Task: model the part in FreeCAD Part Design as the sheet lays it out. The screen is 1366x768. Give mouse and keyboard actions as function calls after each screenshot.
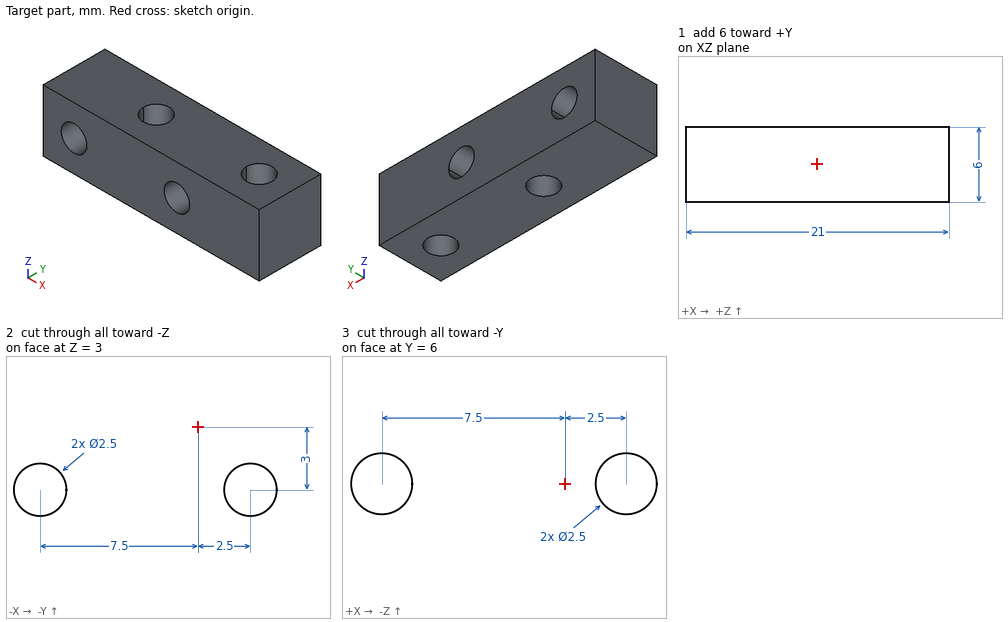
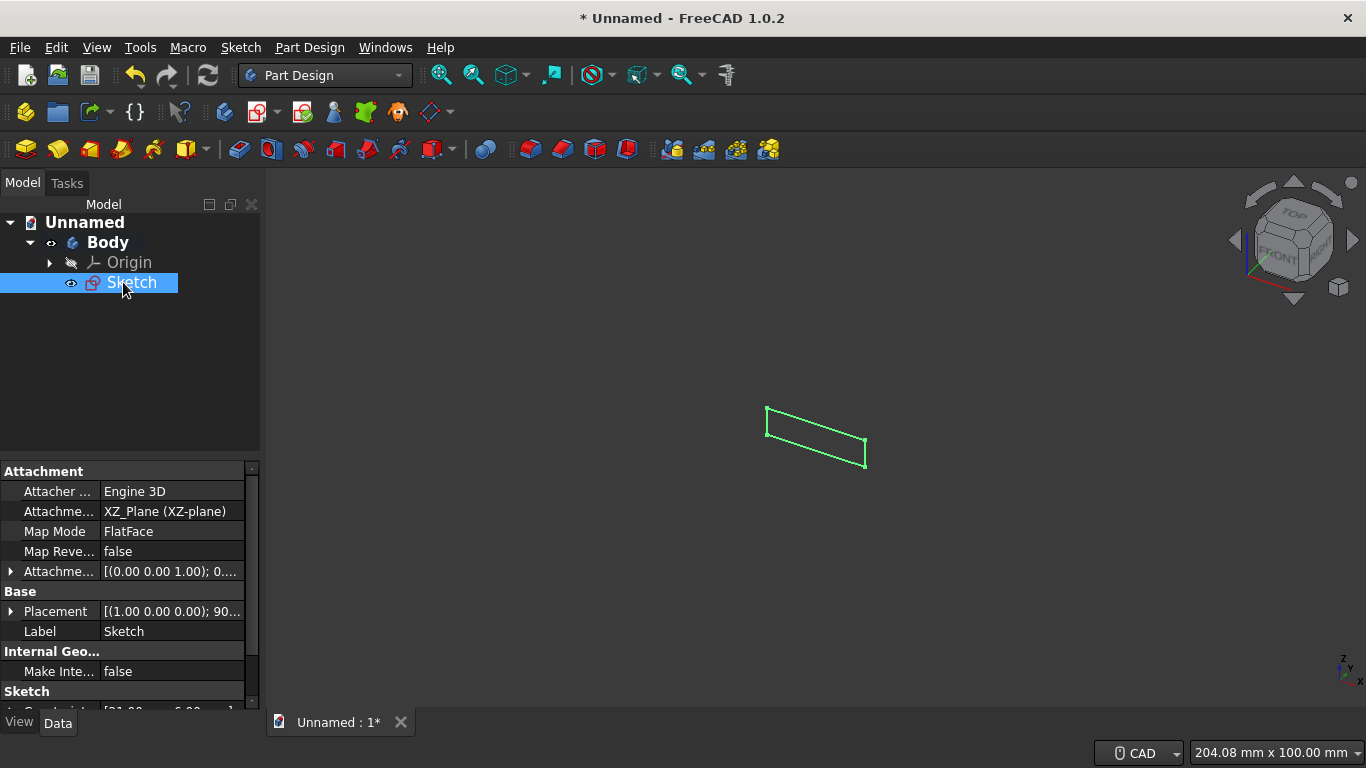
click(26, 150)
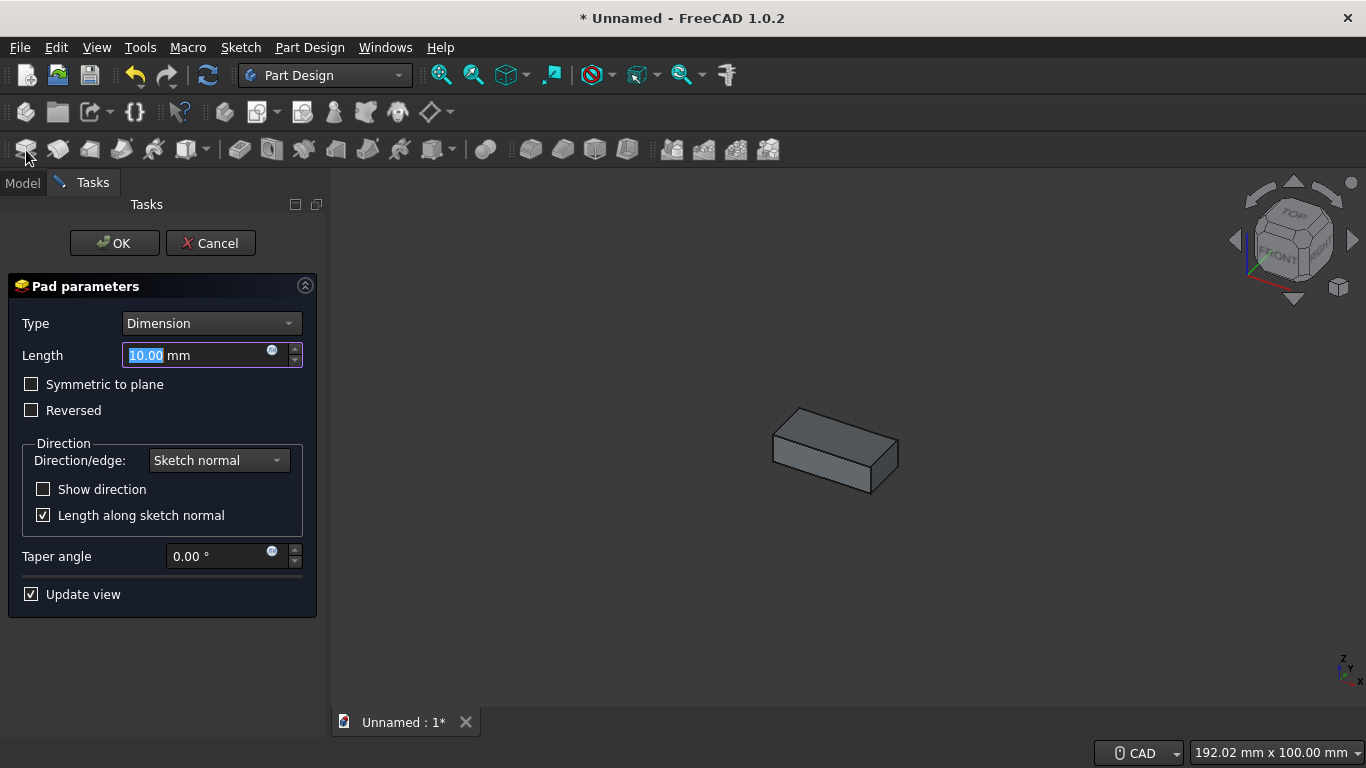
text(6)
key(Tab)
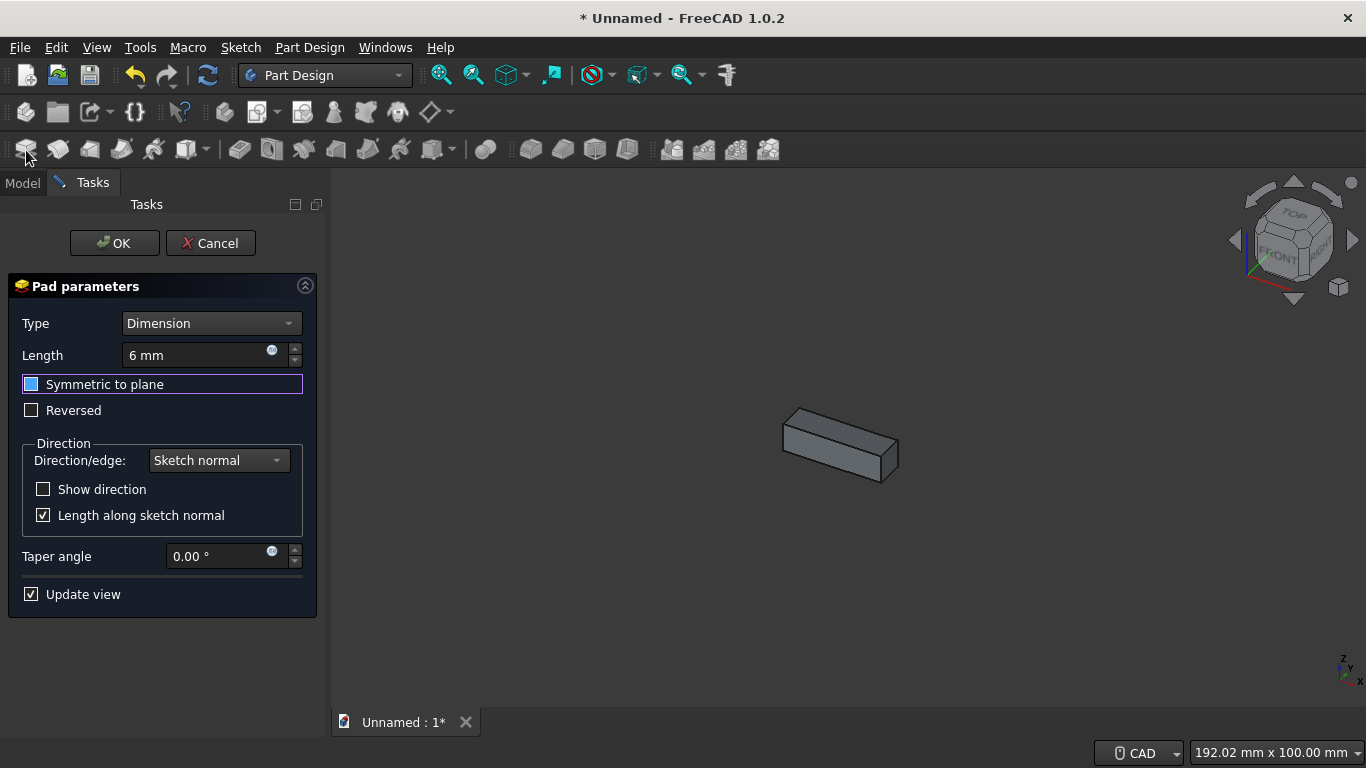
click(30, 410)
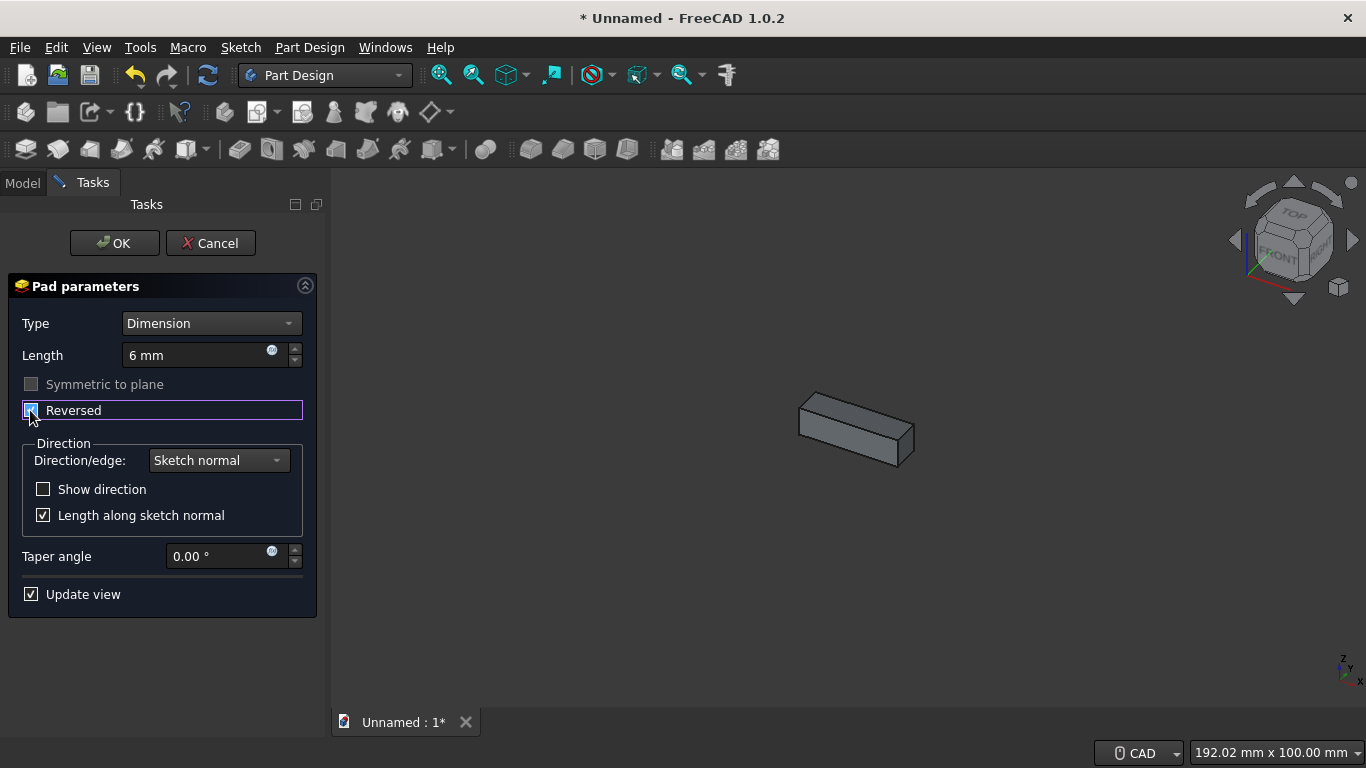
click(115, 243)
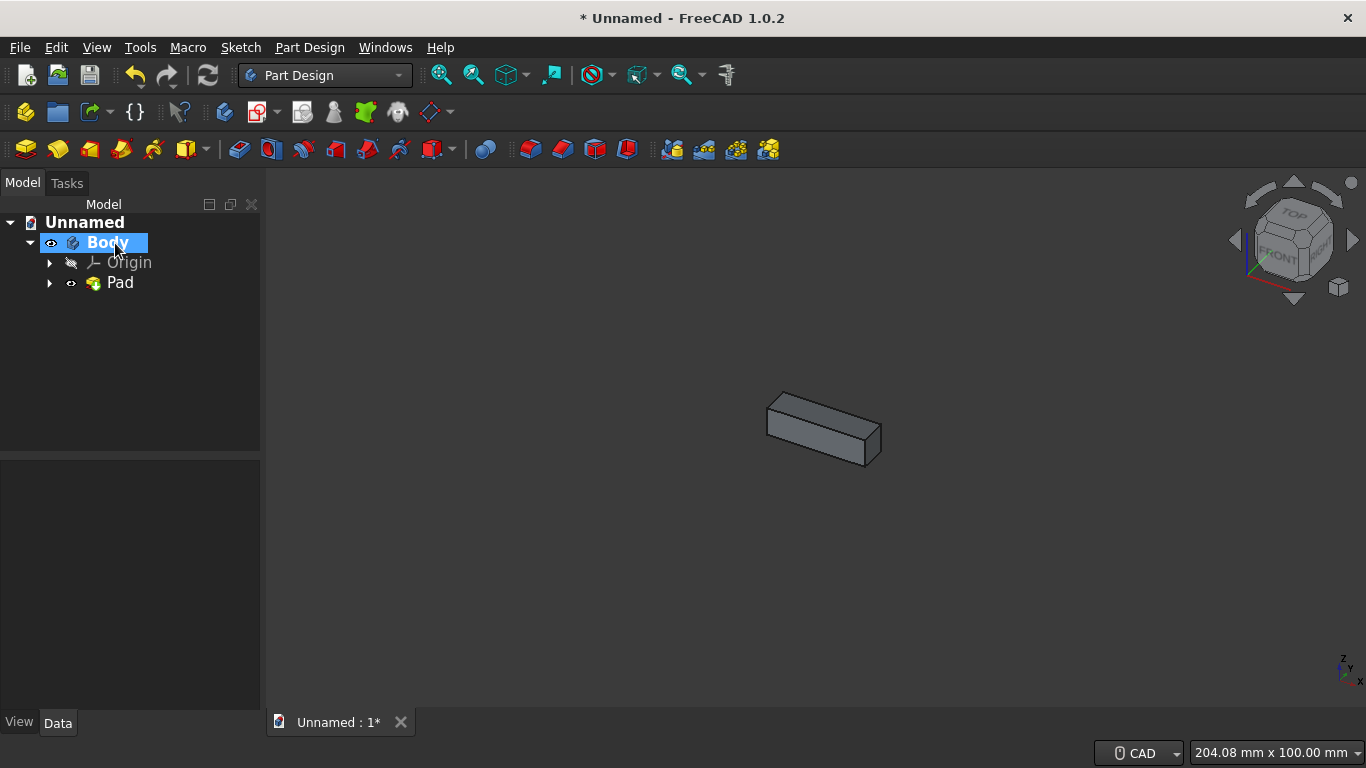
click(442, 76)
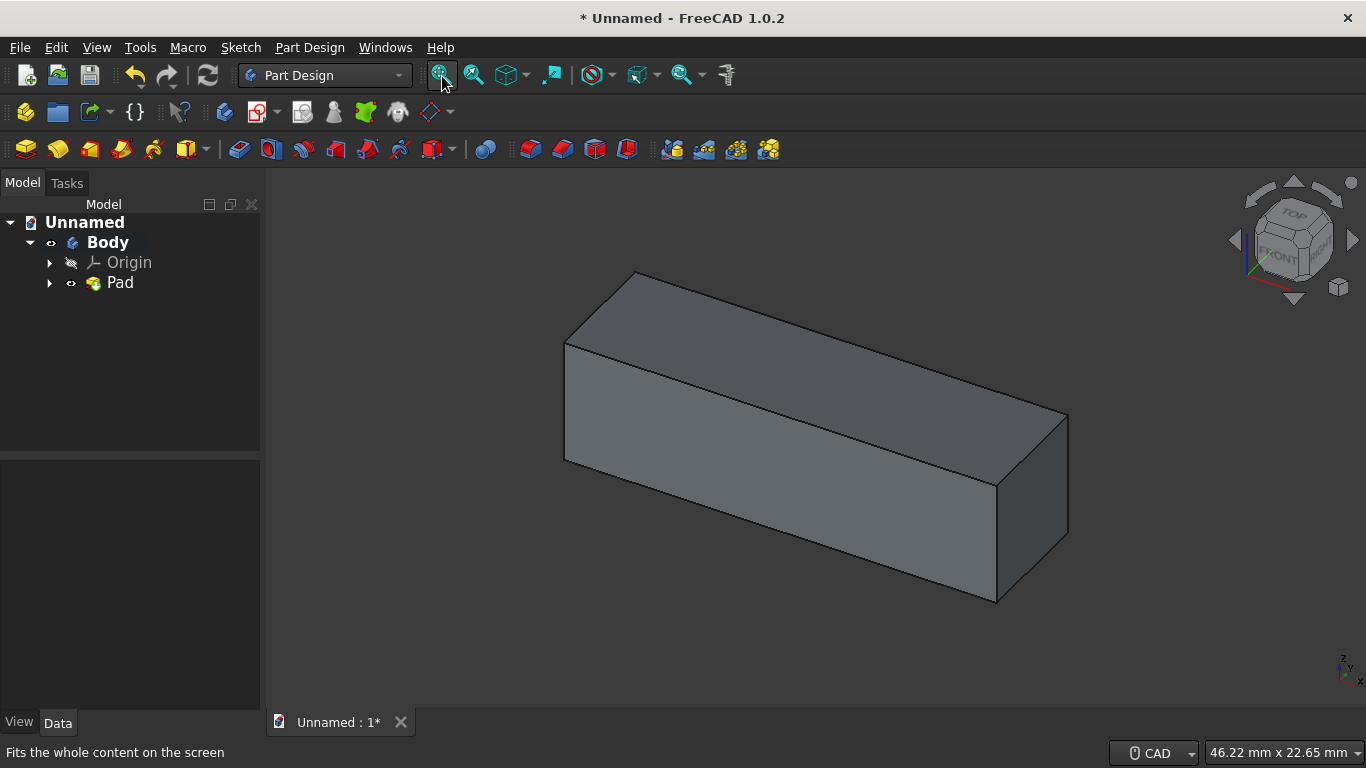
click(940, 419)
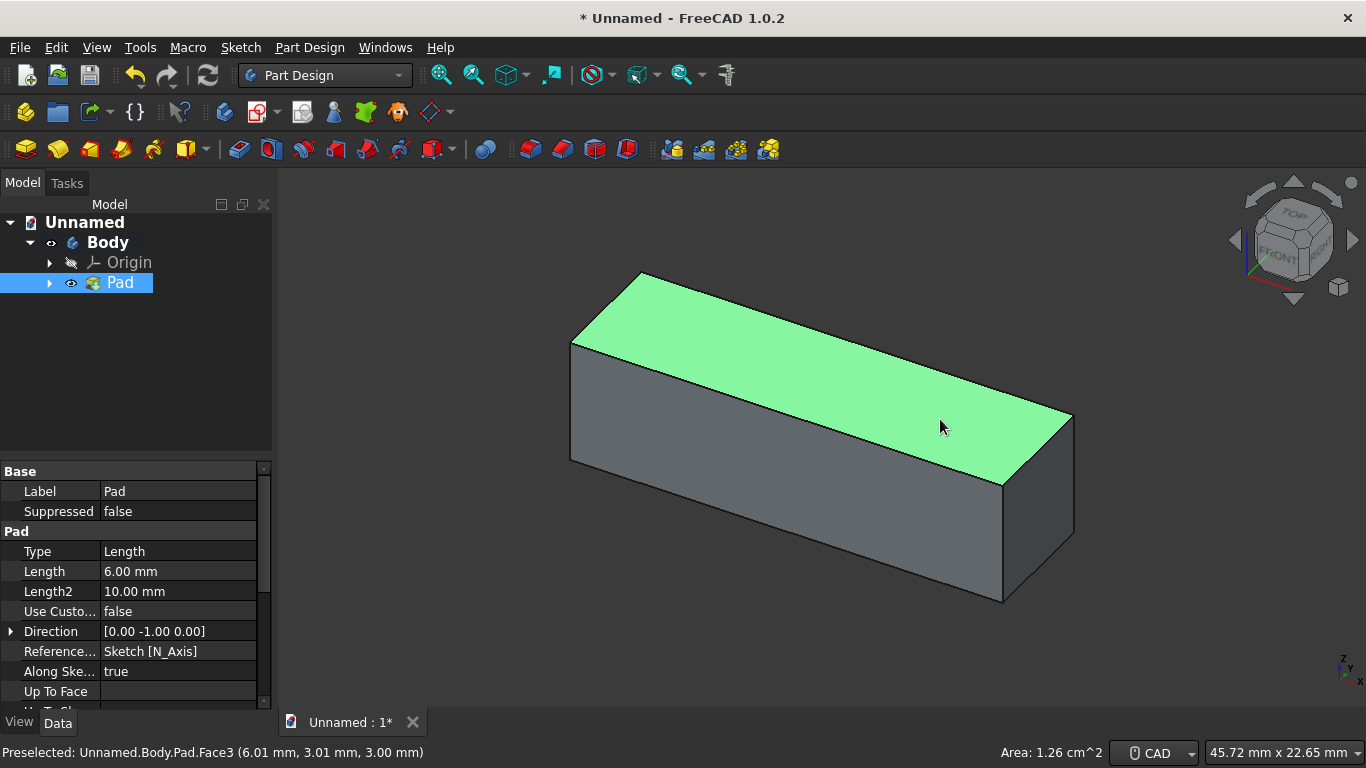
click(258, 112)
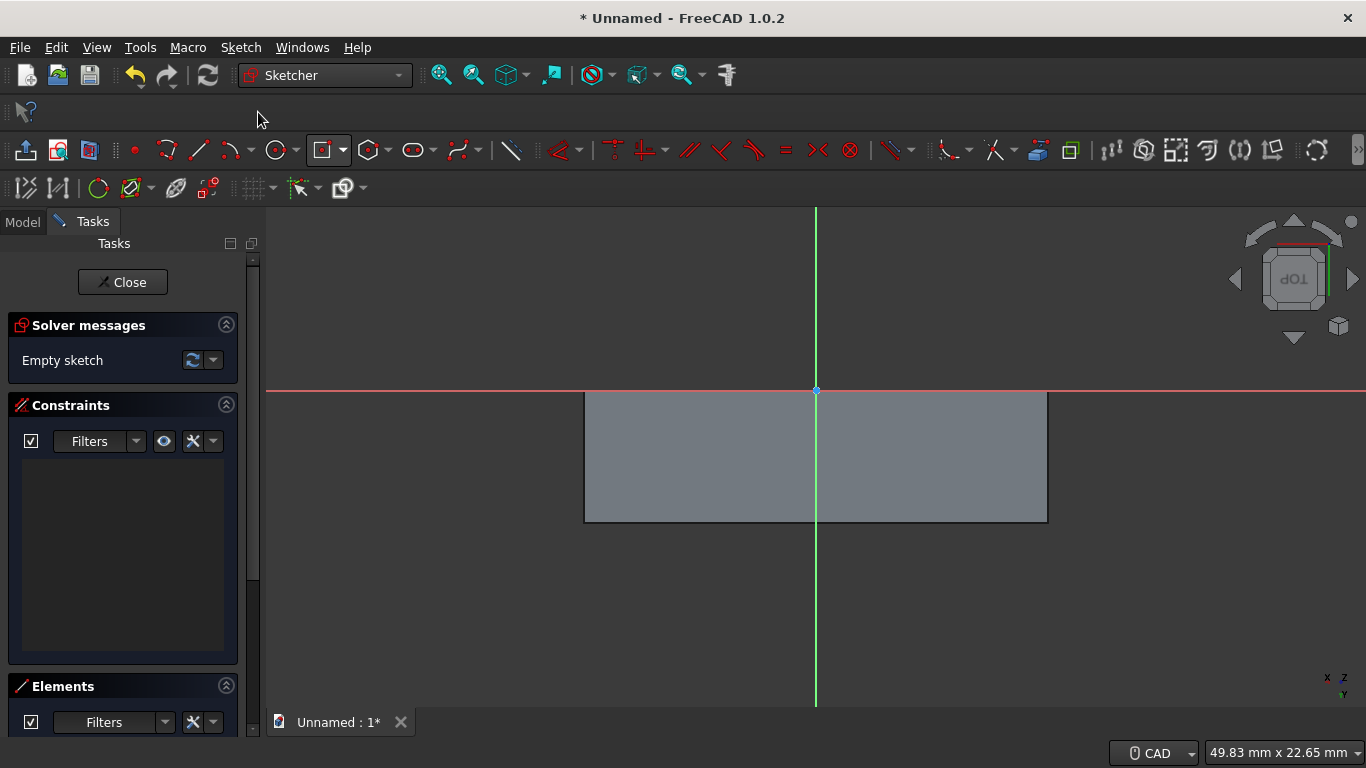
scroll(772, 422, up, 4)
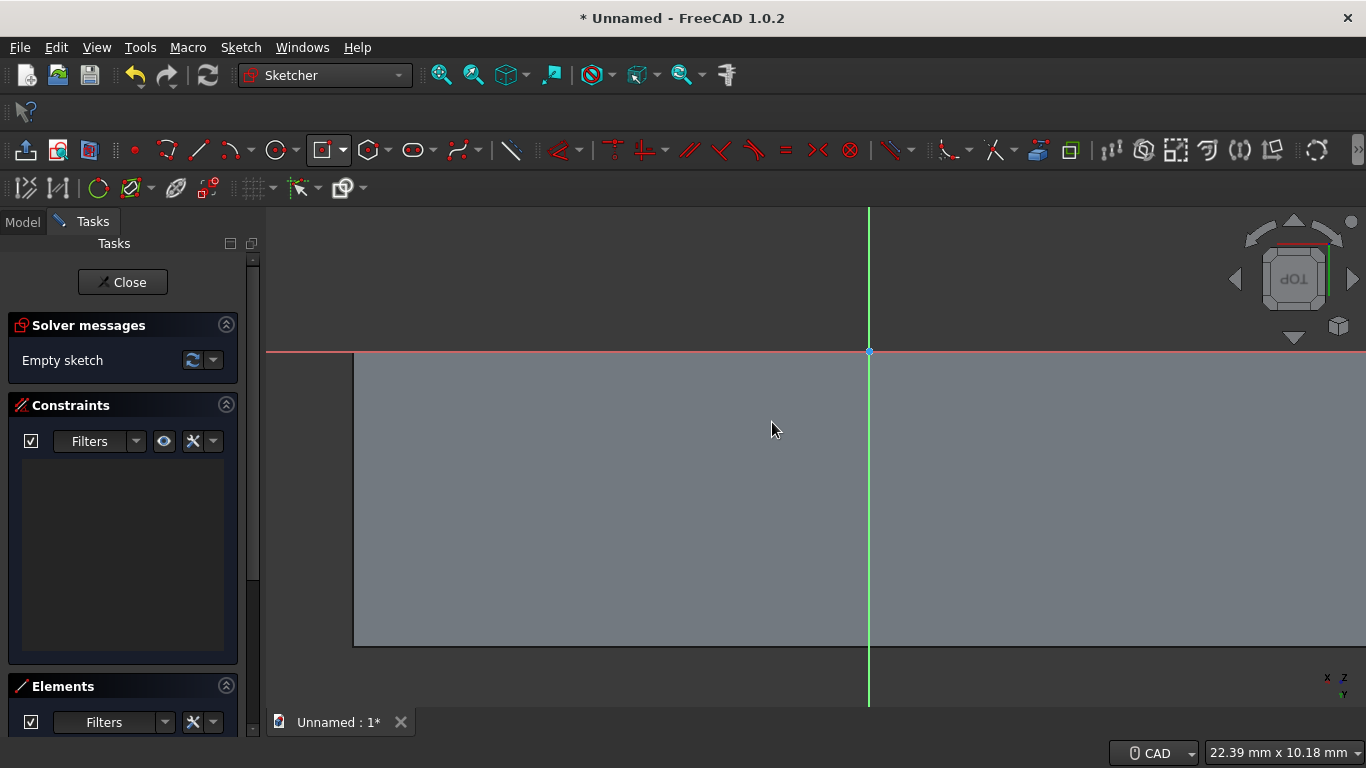
click(276, 150)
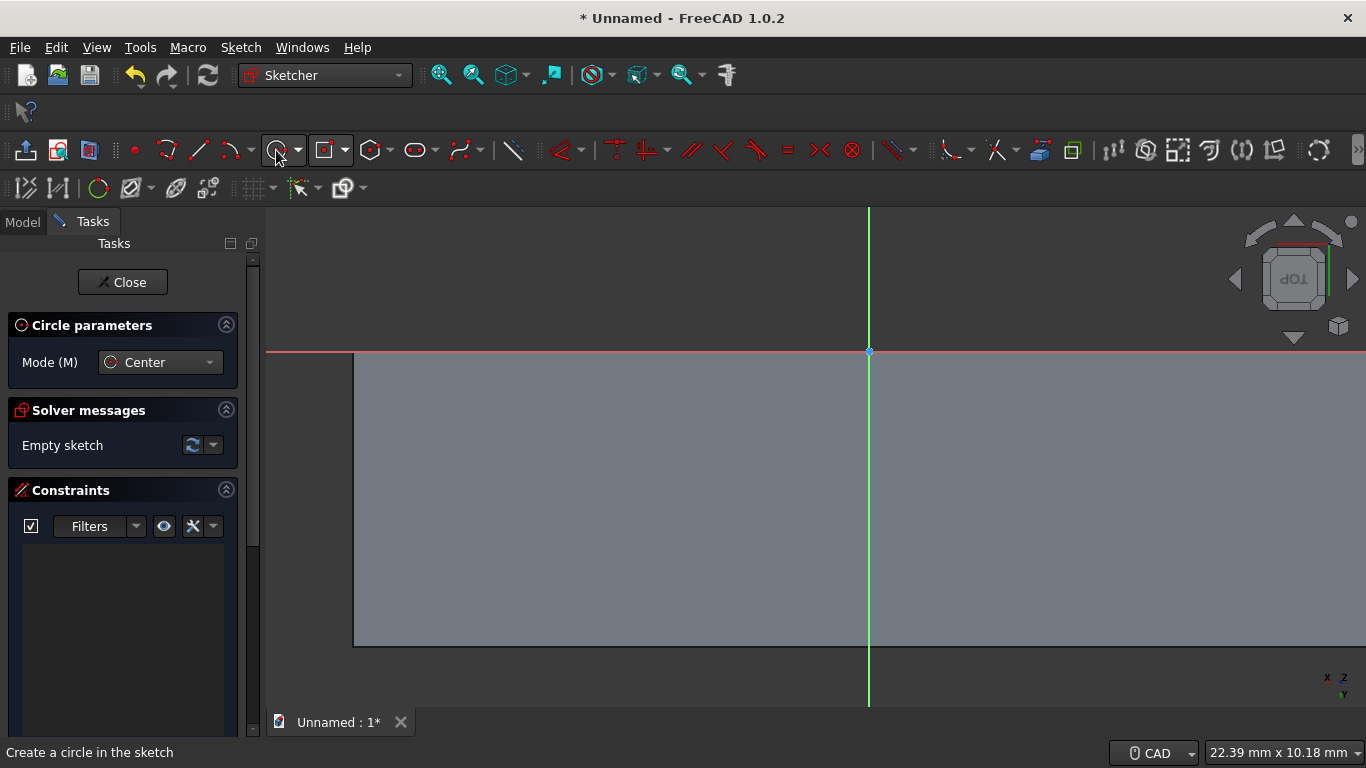
click(992, 499)
move(1036, 456)